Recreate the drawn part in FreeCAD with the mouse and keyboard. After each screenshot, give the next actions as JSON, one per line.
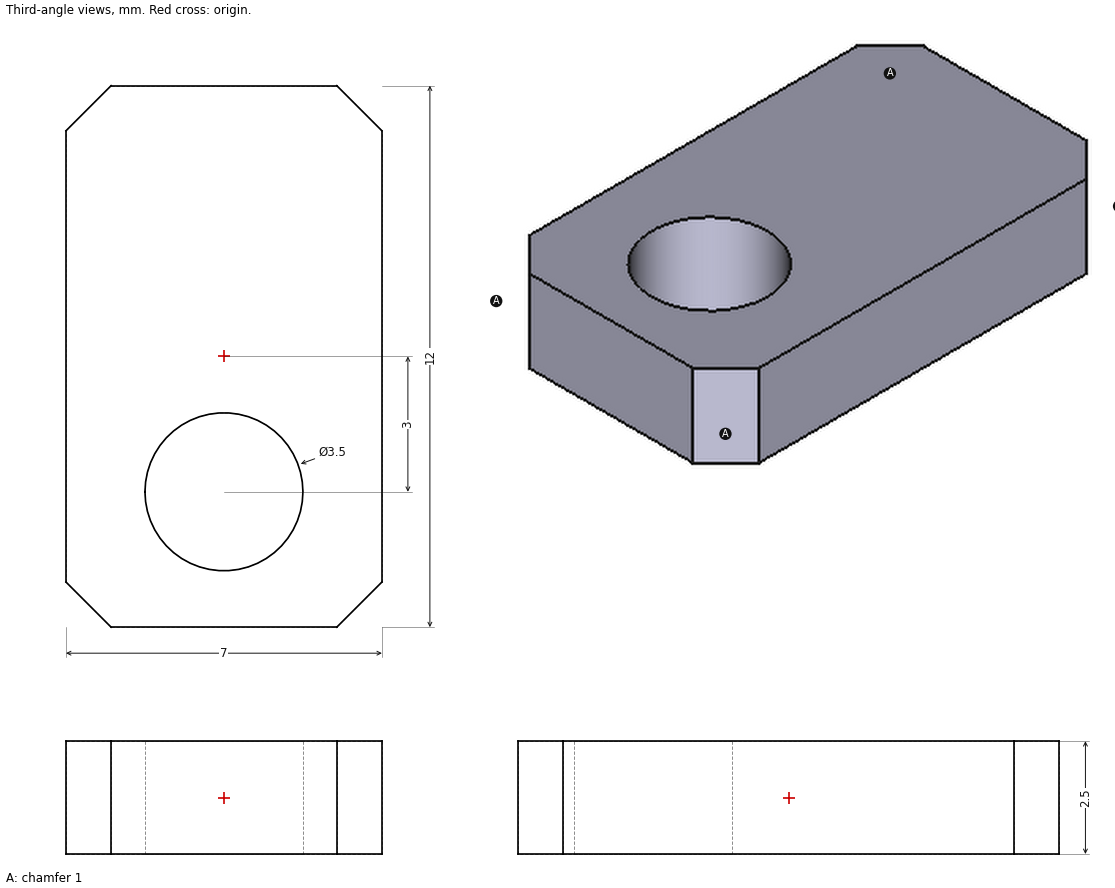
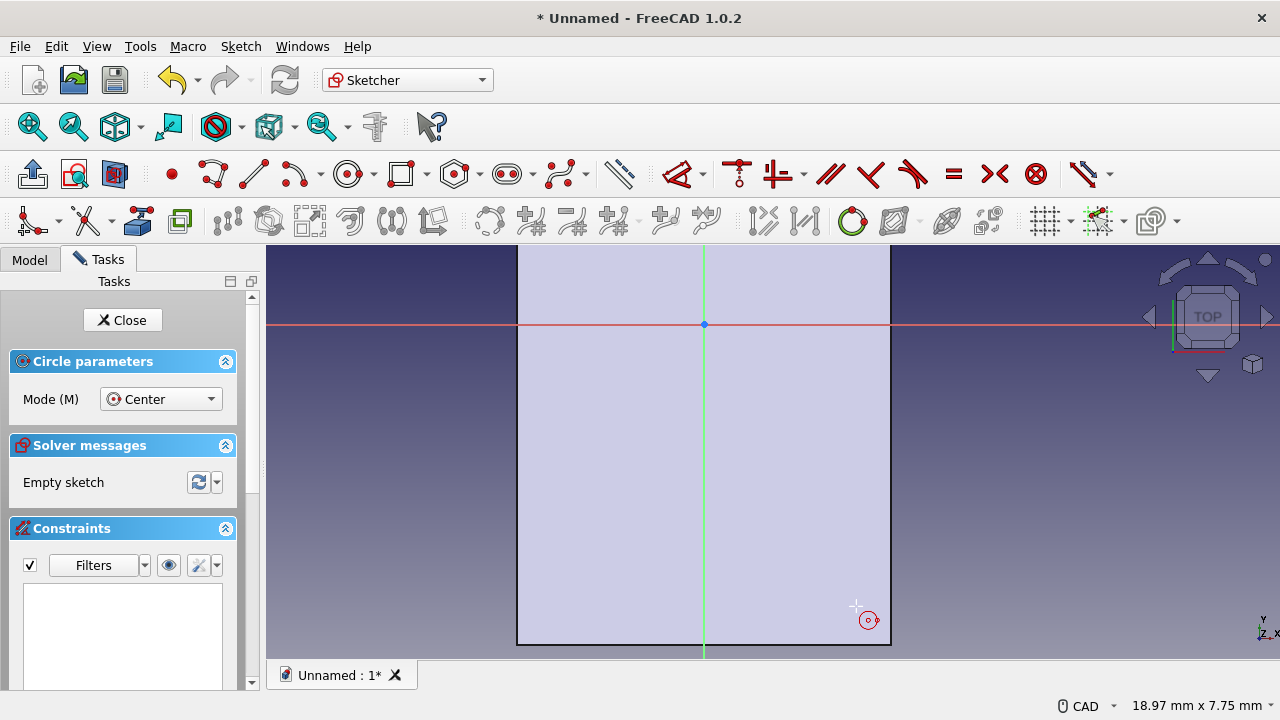
{"action": "left_click", "coordinate": [704, 485]}
{"action": "left_click", "coordinate": [770, 419]}
{"action": "key", "text": "Escape"}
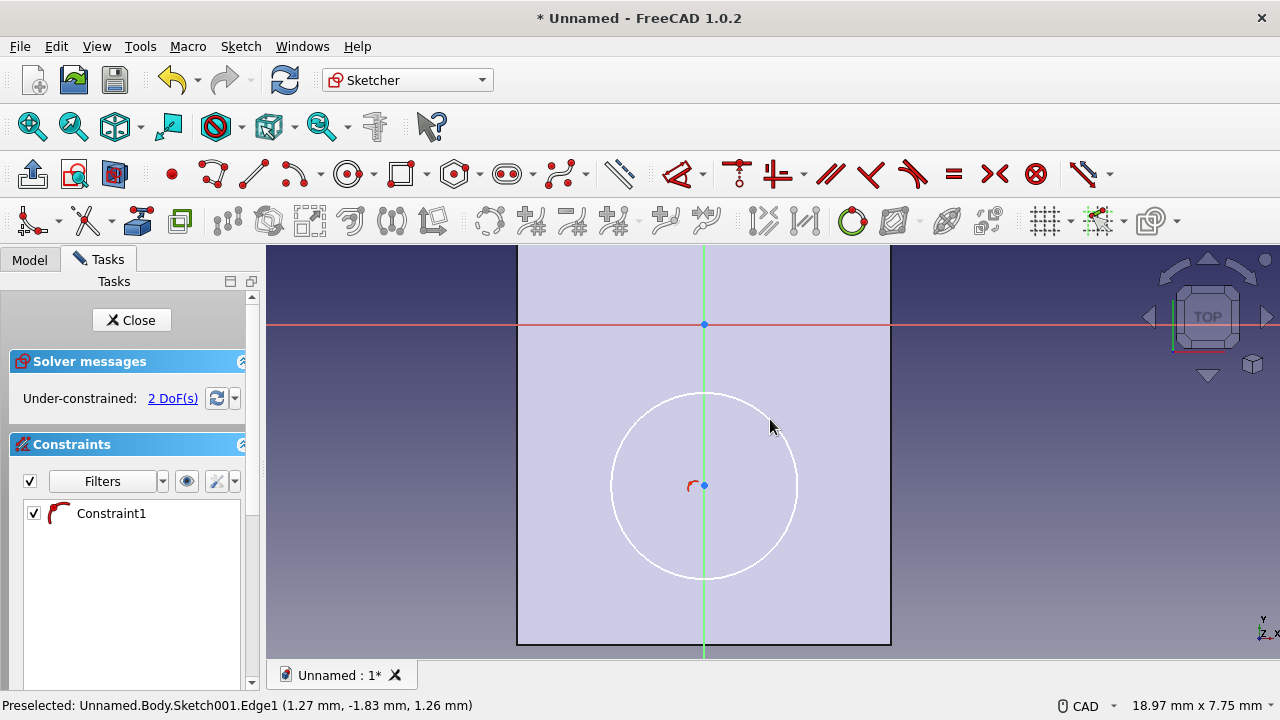
{"action": "left_click", "coordinate": [676, 174]}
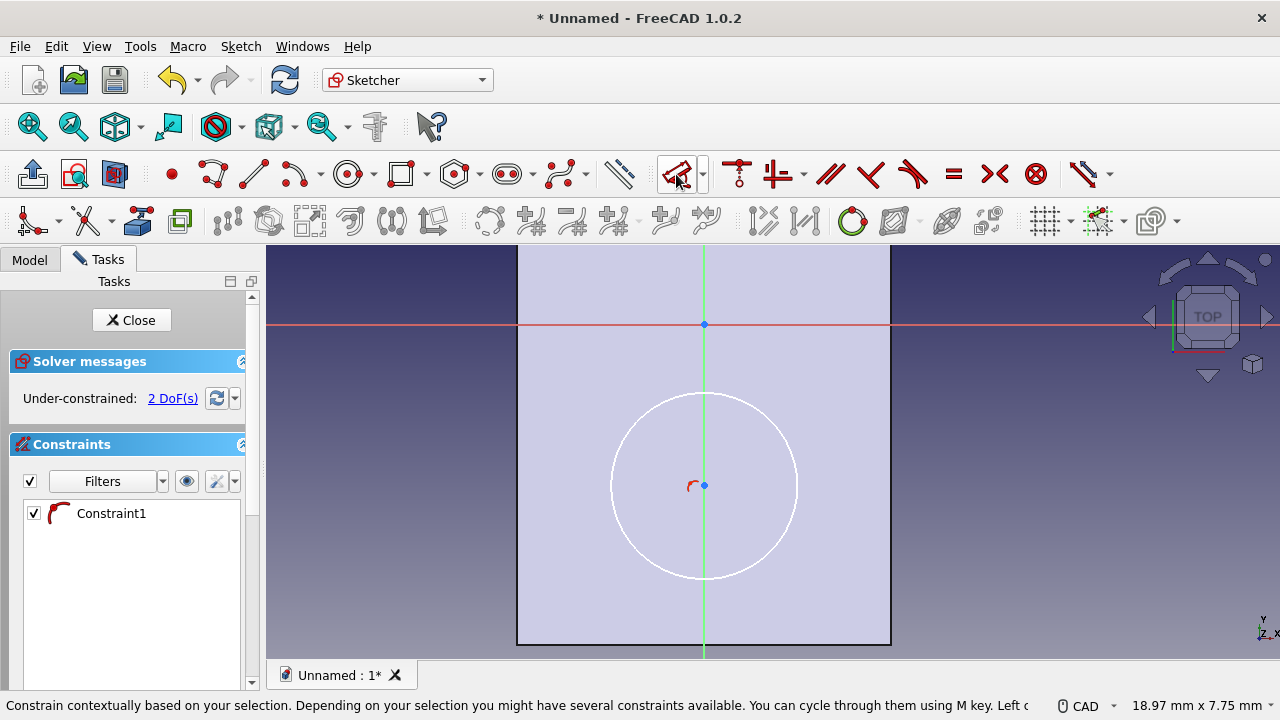
{"action": "left_click", "coordinate": [770, 420]}
{"action": "left_click", "coordinate": [793, 397]}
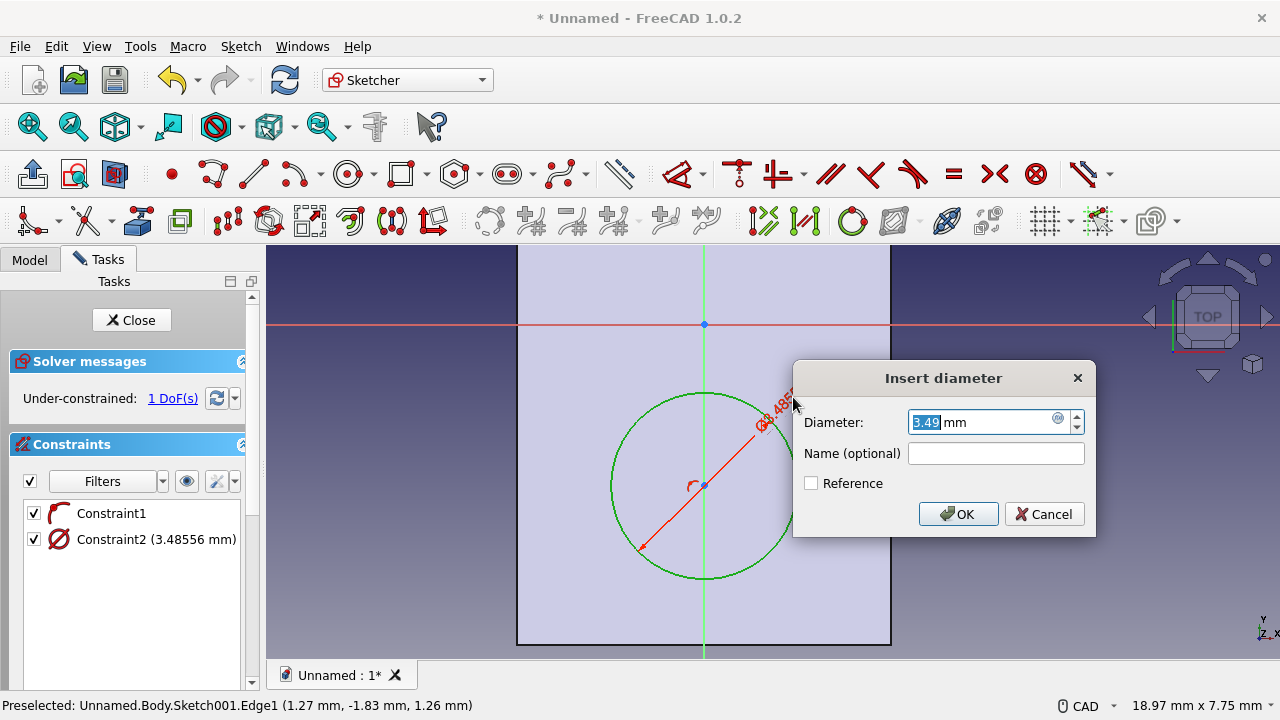
{"action": "type", "text": "3.5"}
{"action": "key", "text": "Return"}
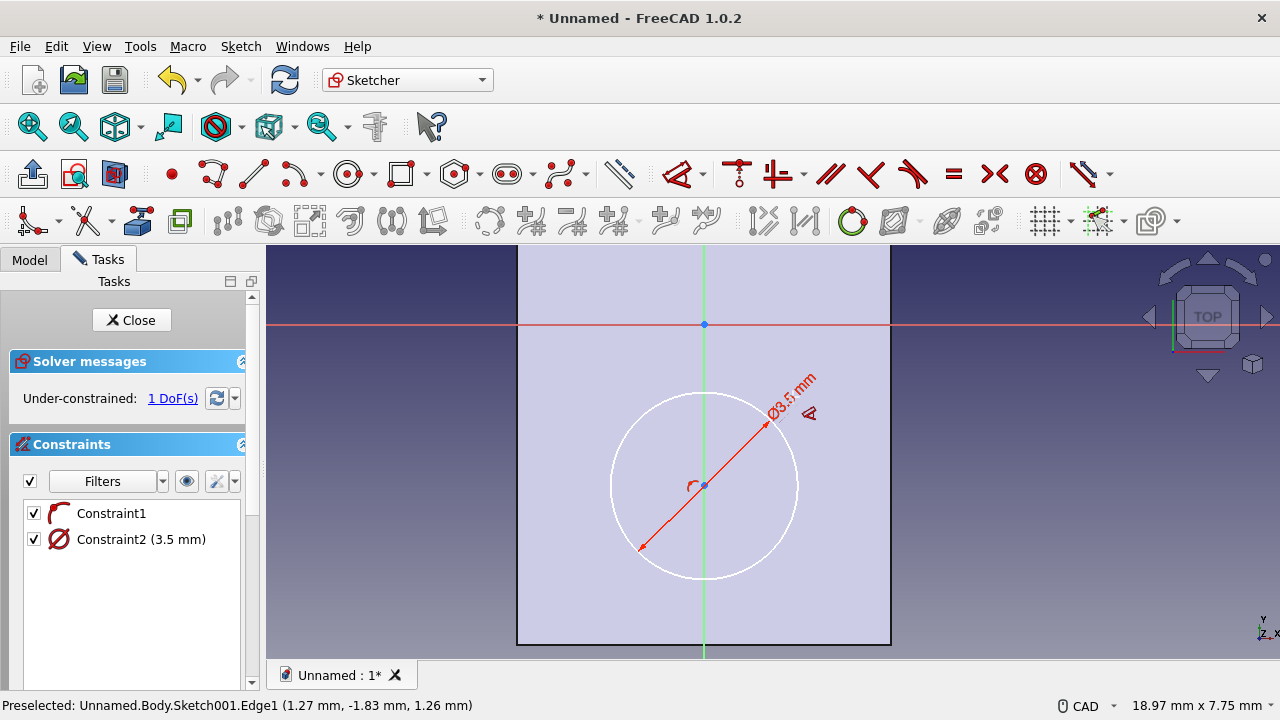
{"action": "left_click", "coordinate": [704, 486]}
{"action": "left_click", "coordinate": [738, 368]}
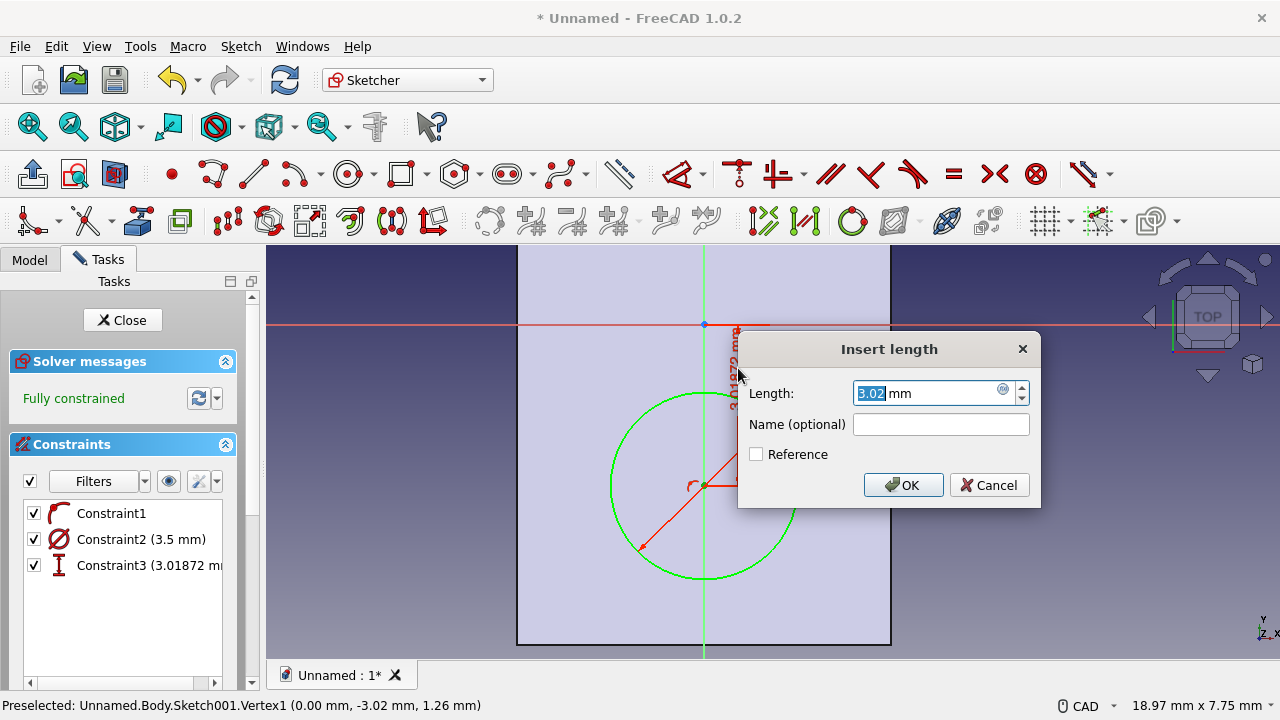
{"action": "type", "text": "3"}
{"action": "key", "text": "Return"}
{"action": "key", "text": "Escape"}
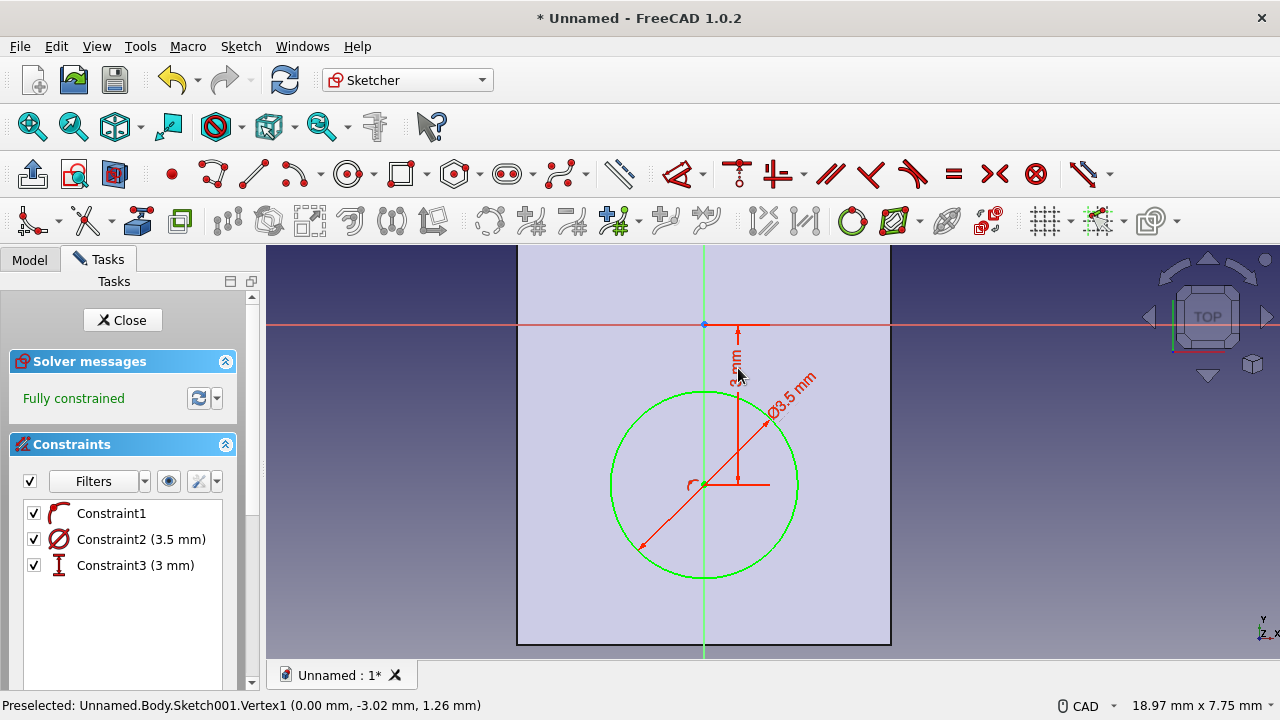
{"action": "left_click", "coordinate": [123, 320]}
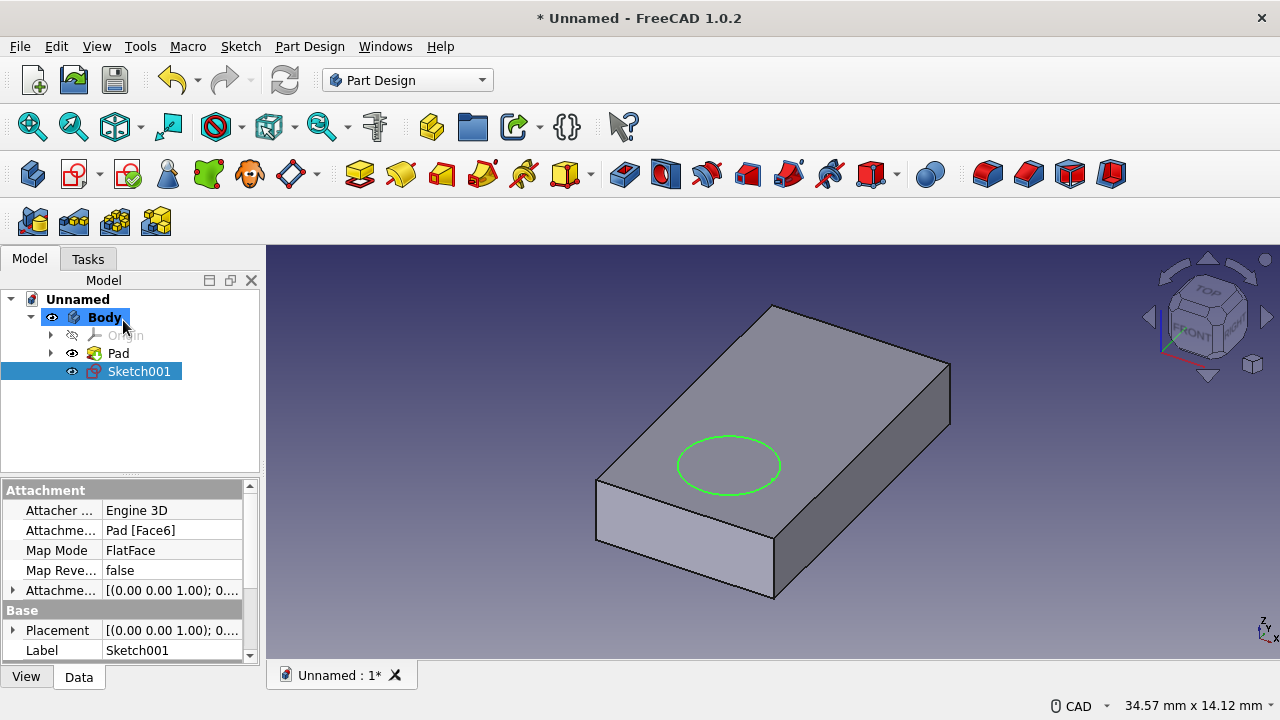
{"action": "left_click", "coordinate": [625, 174]}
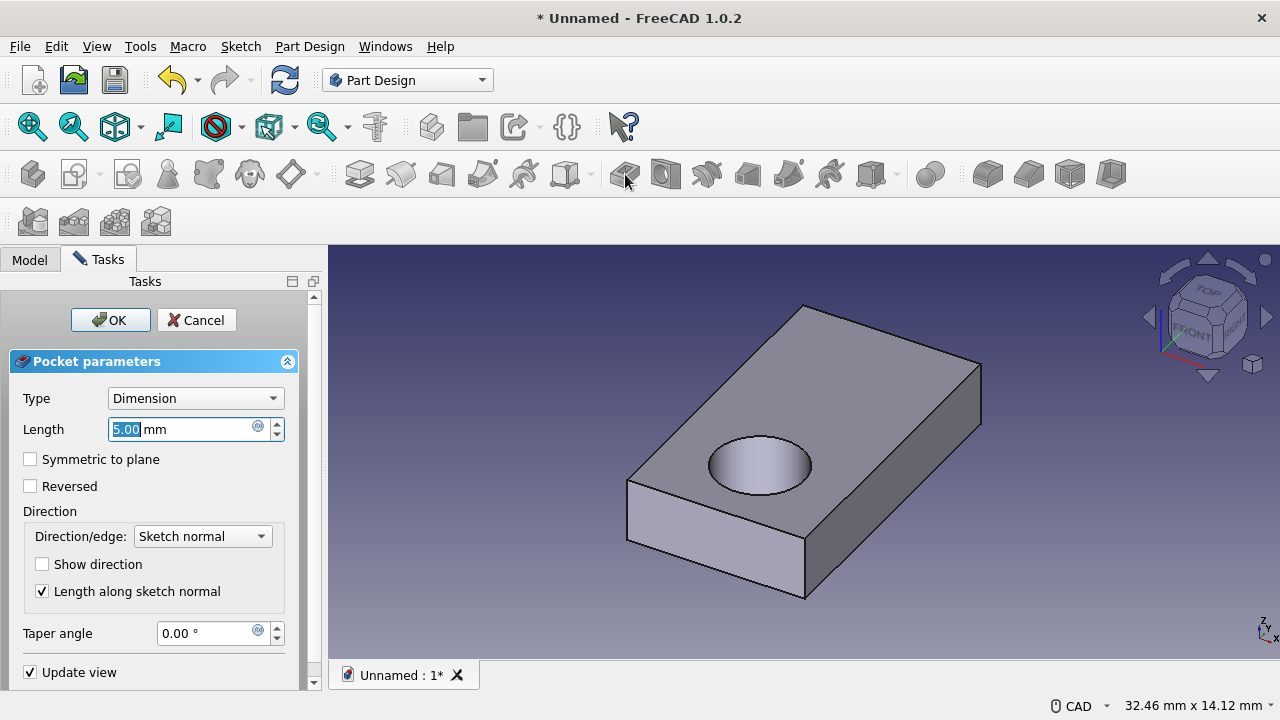
{"action": "left_click", "coordinate": [196, 398]}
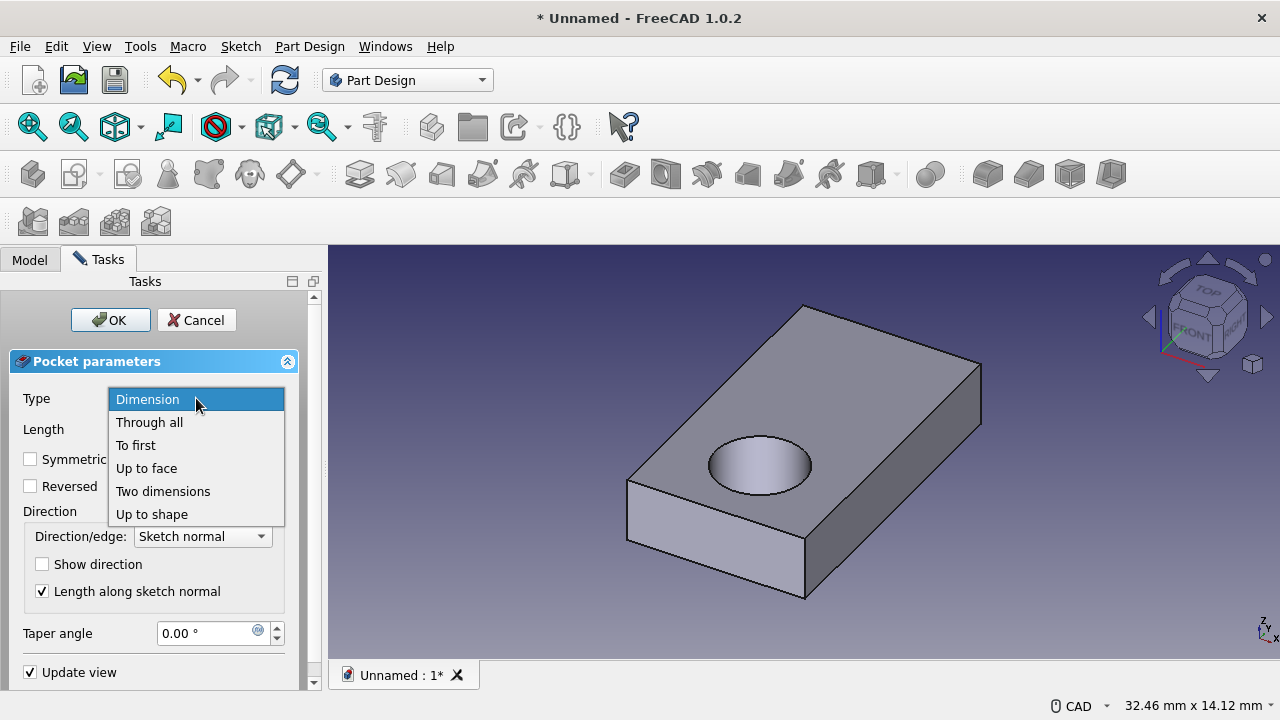
{"action": "left_click", "coordinate": [194, 422]}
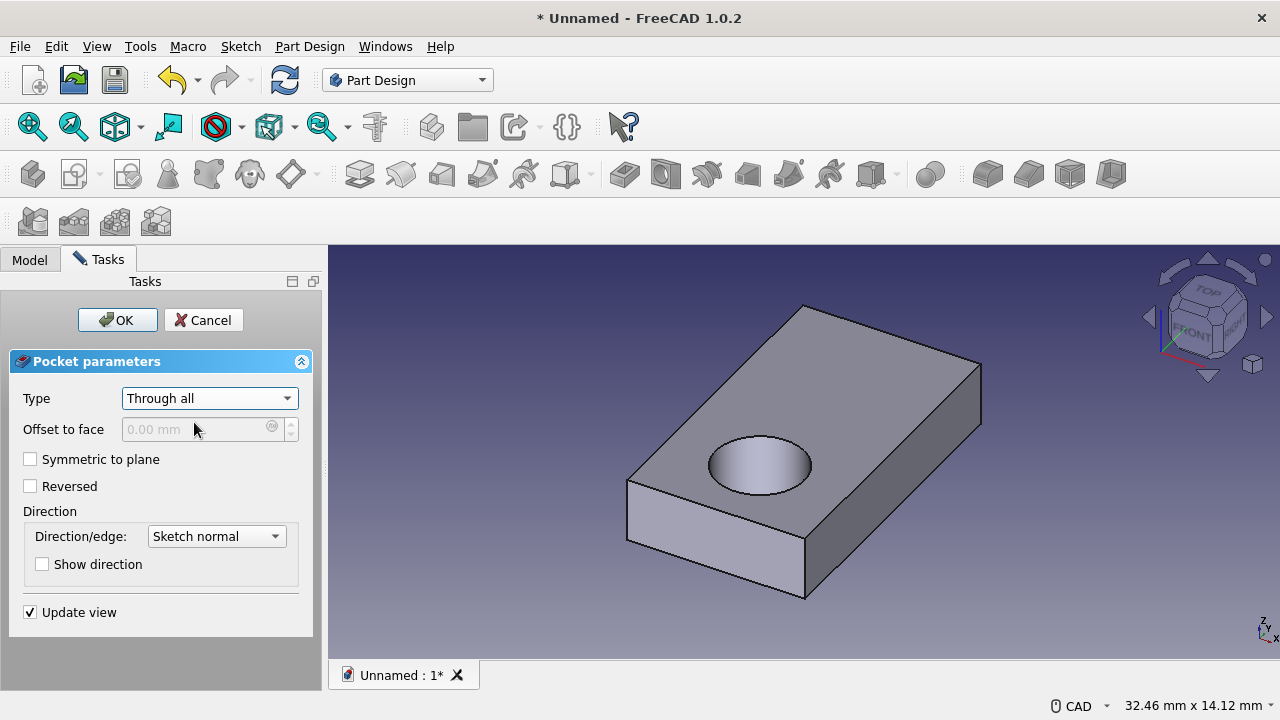
{"action": "left_click", "coordinate": [118, 320]}